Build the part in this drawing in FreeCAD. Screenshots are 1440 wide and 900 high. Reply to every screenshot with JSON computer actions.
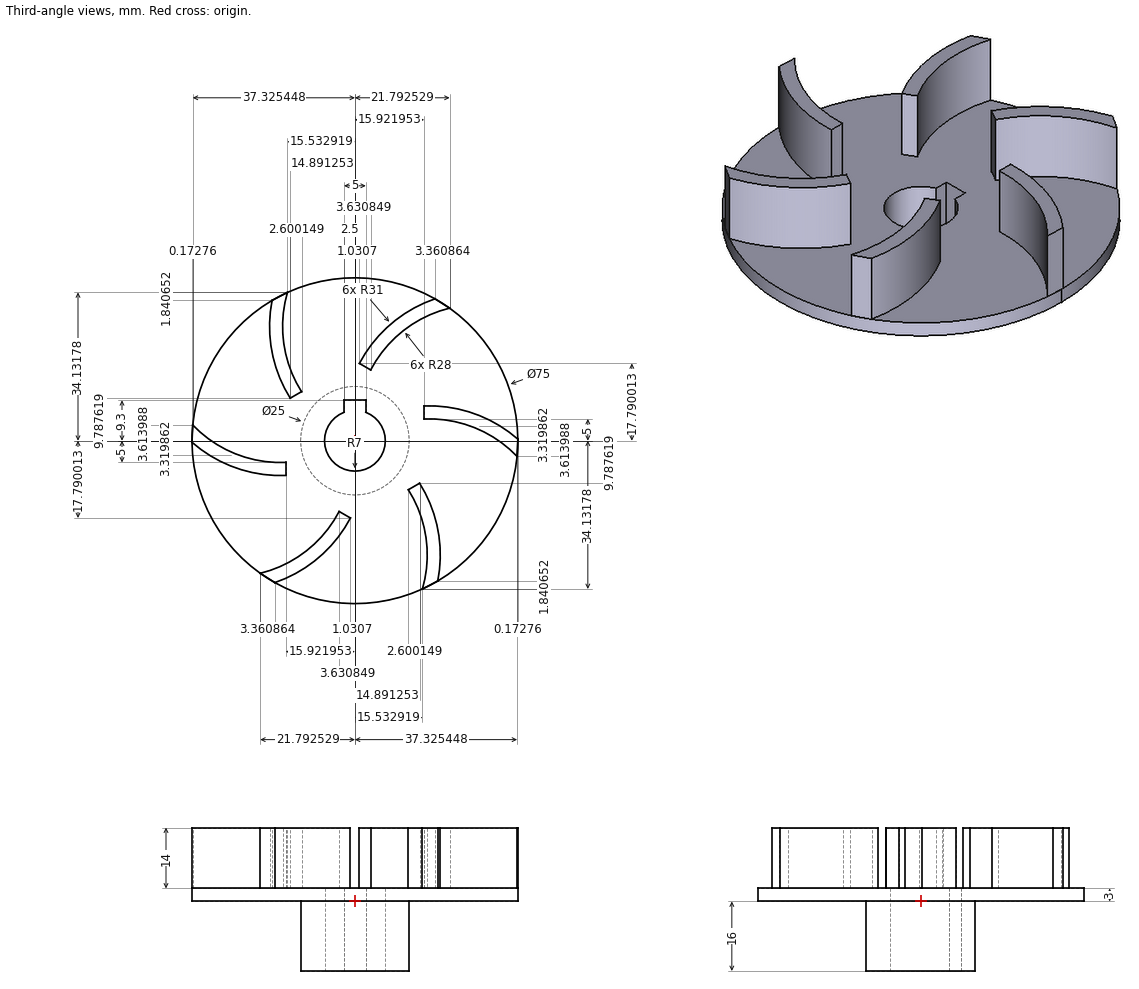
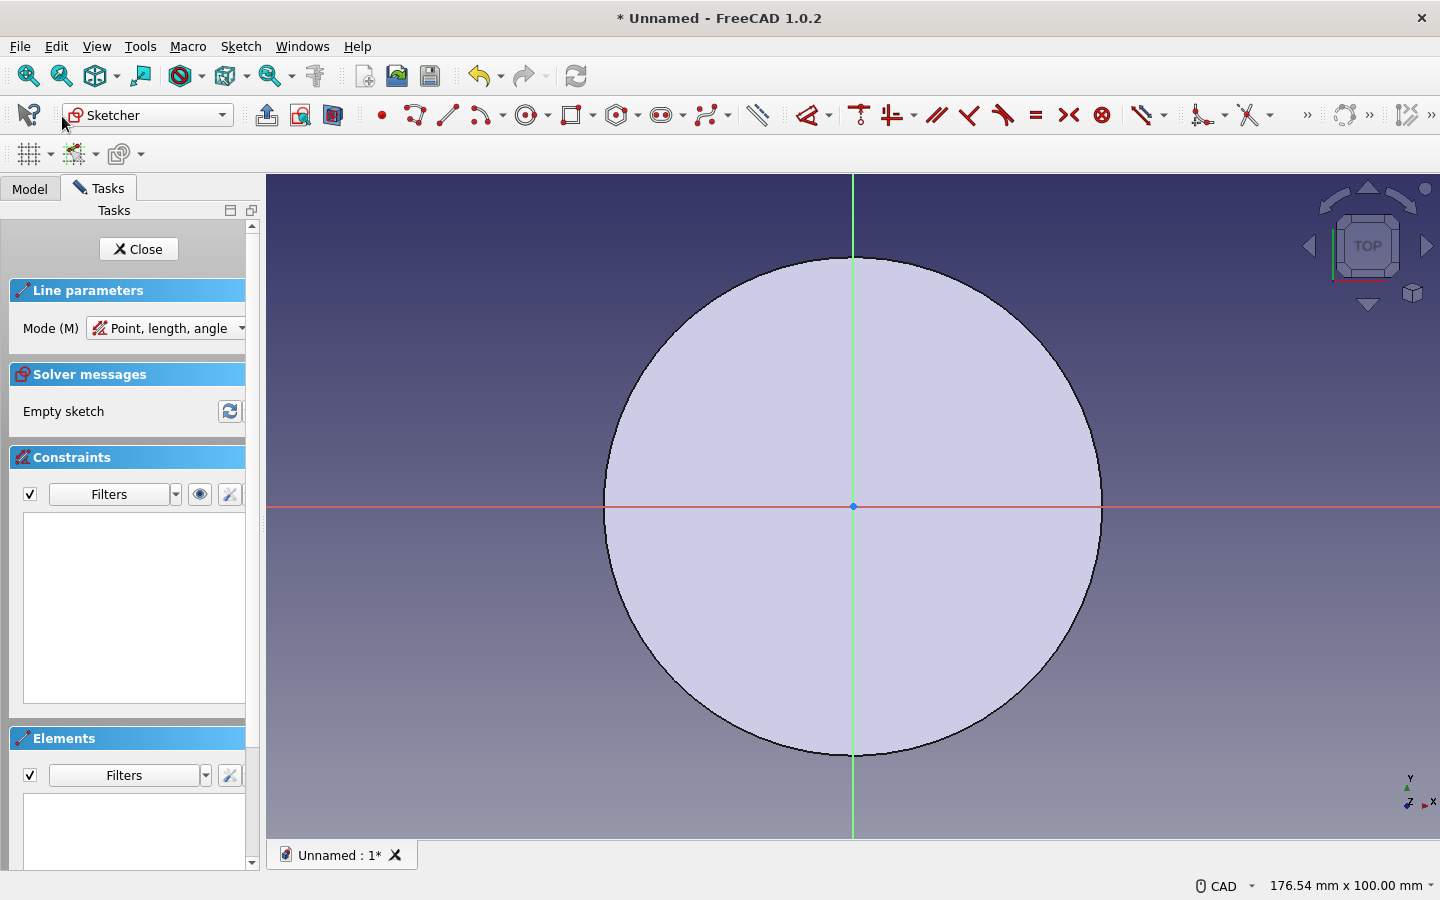
{"action": "left_click", "coordinate": [998, 304]}
{"action": "left_click", "coordinate": [976, 289]}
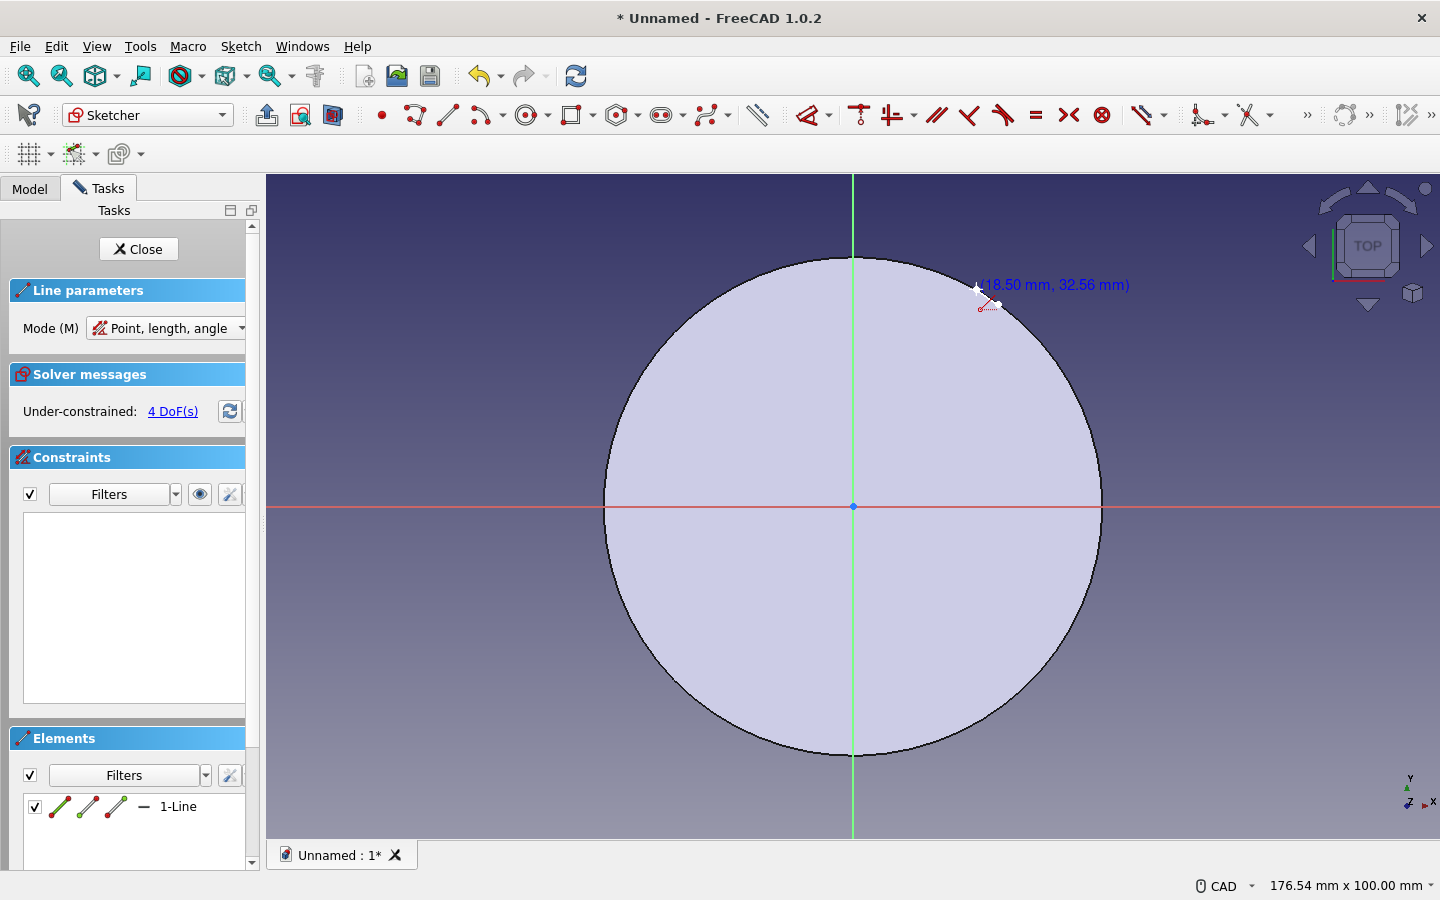
{"action": "scroll", "coordinate": [860, 388], "scroll_direction": "up", "scroll_amount": 5}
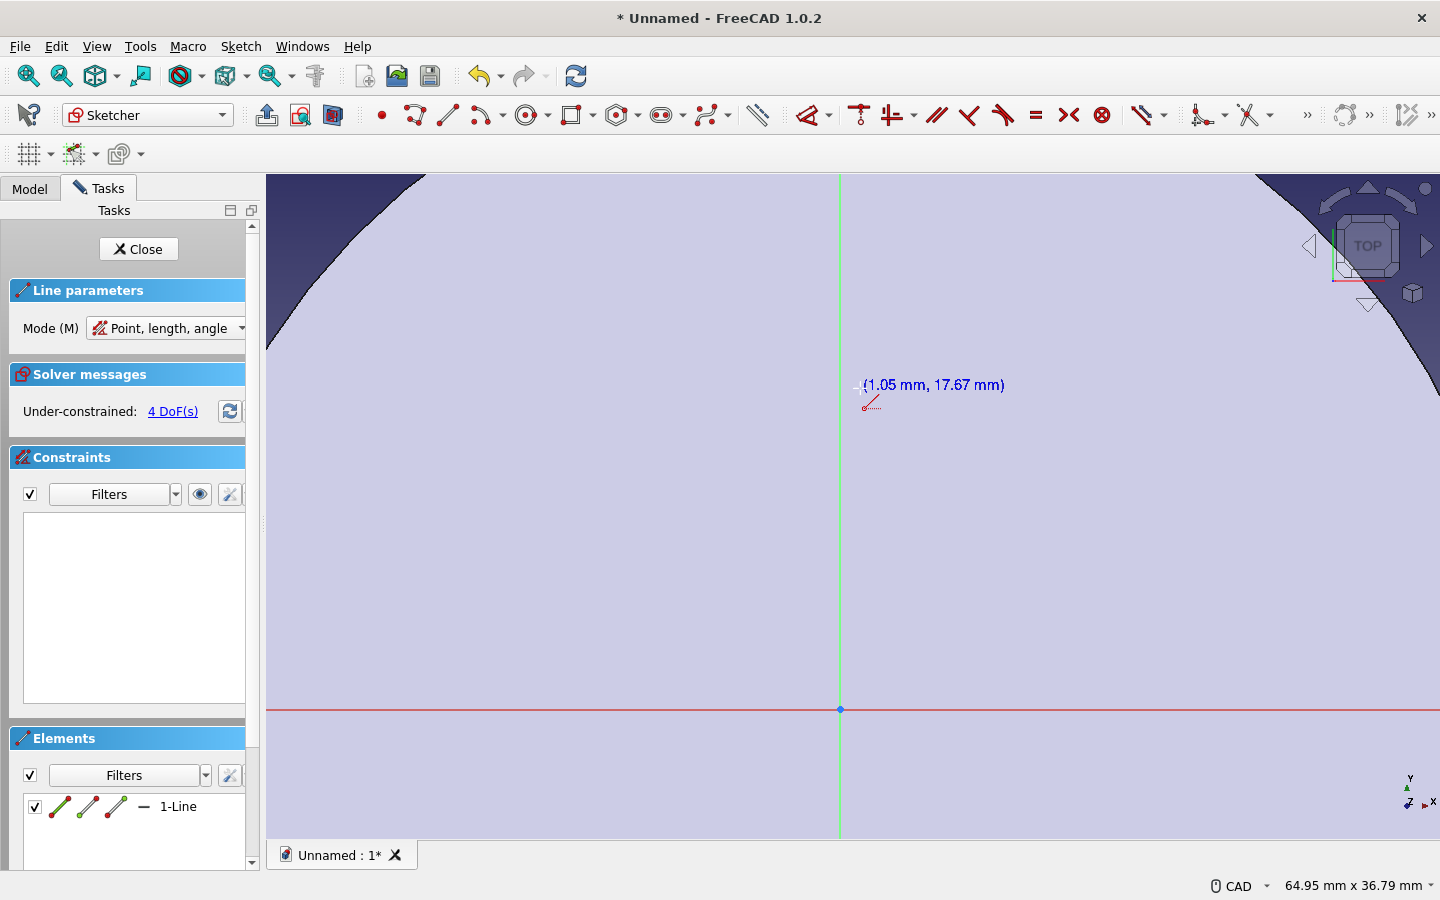
{"action": "left_click", "coordinate": [859, 388]}
{"action": "left_click", "coordinate": [906, 415]}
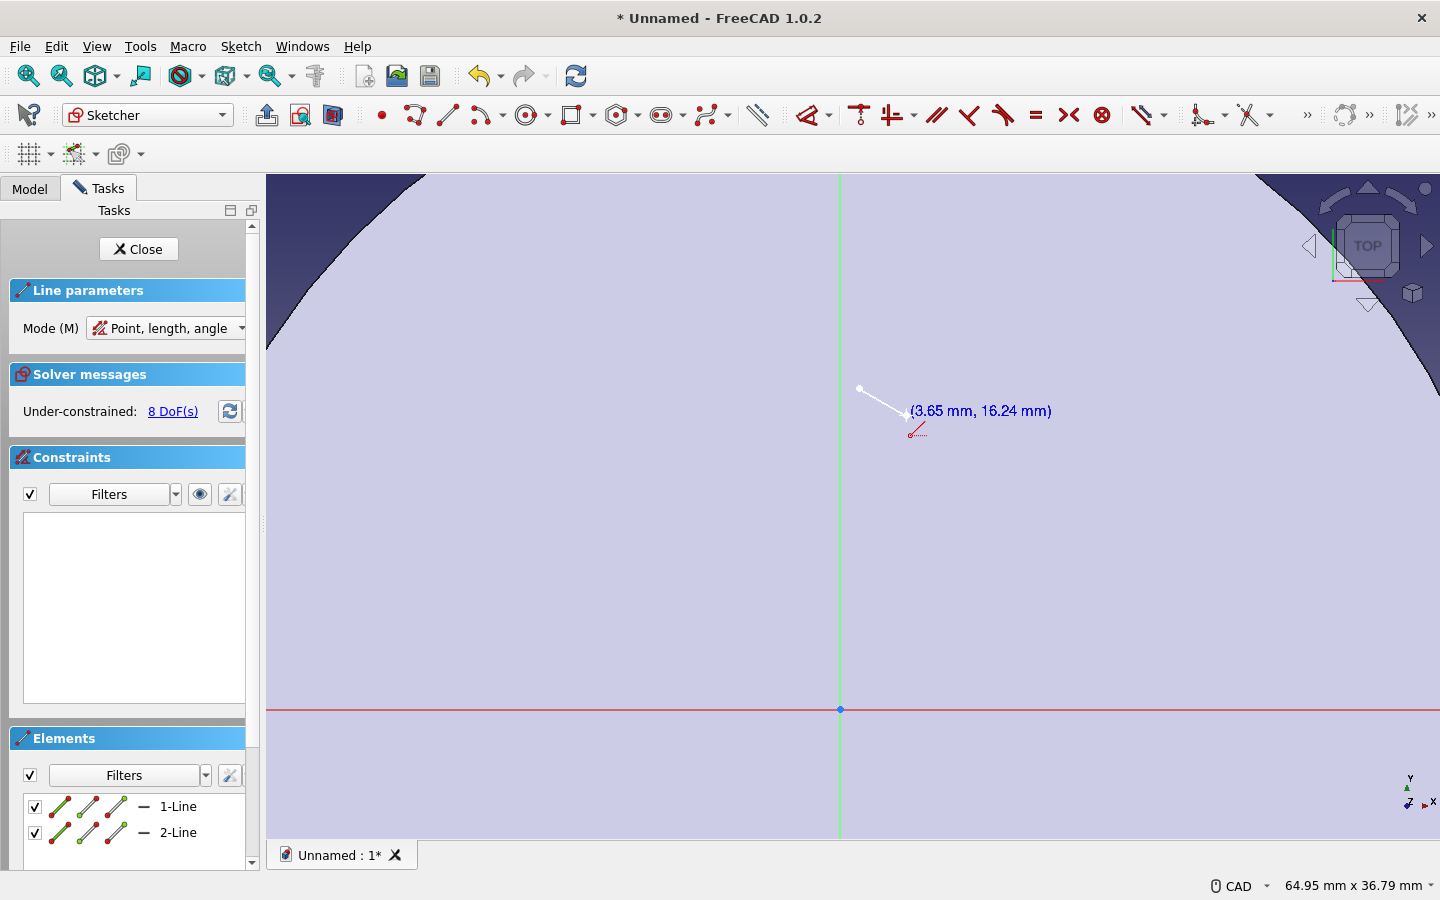
{"action": "key", "text": "g 3 a"}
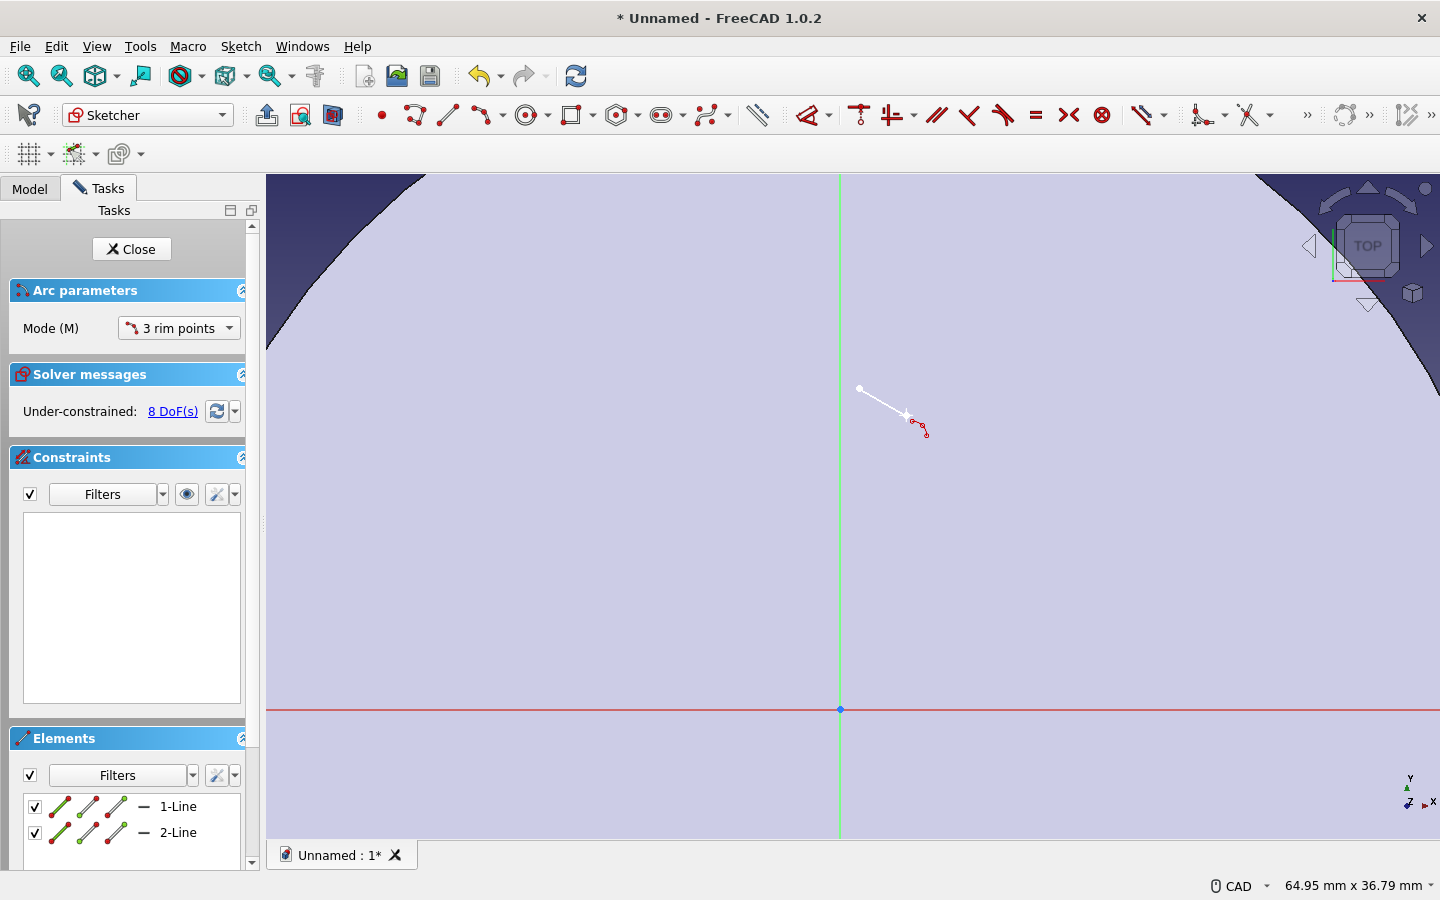
{"action": "scroll", "coordinate": [752, 388], "scroll_direction": "down", "scroll_amount": 5}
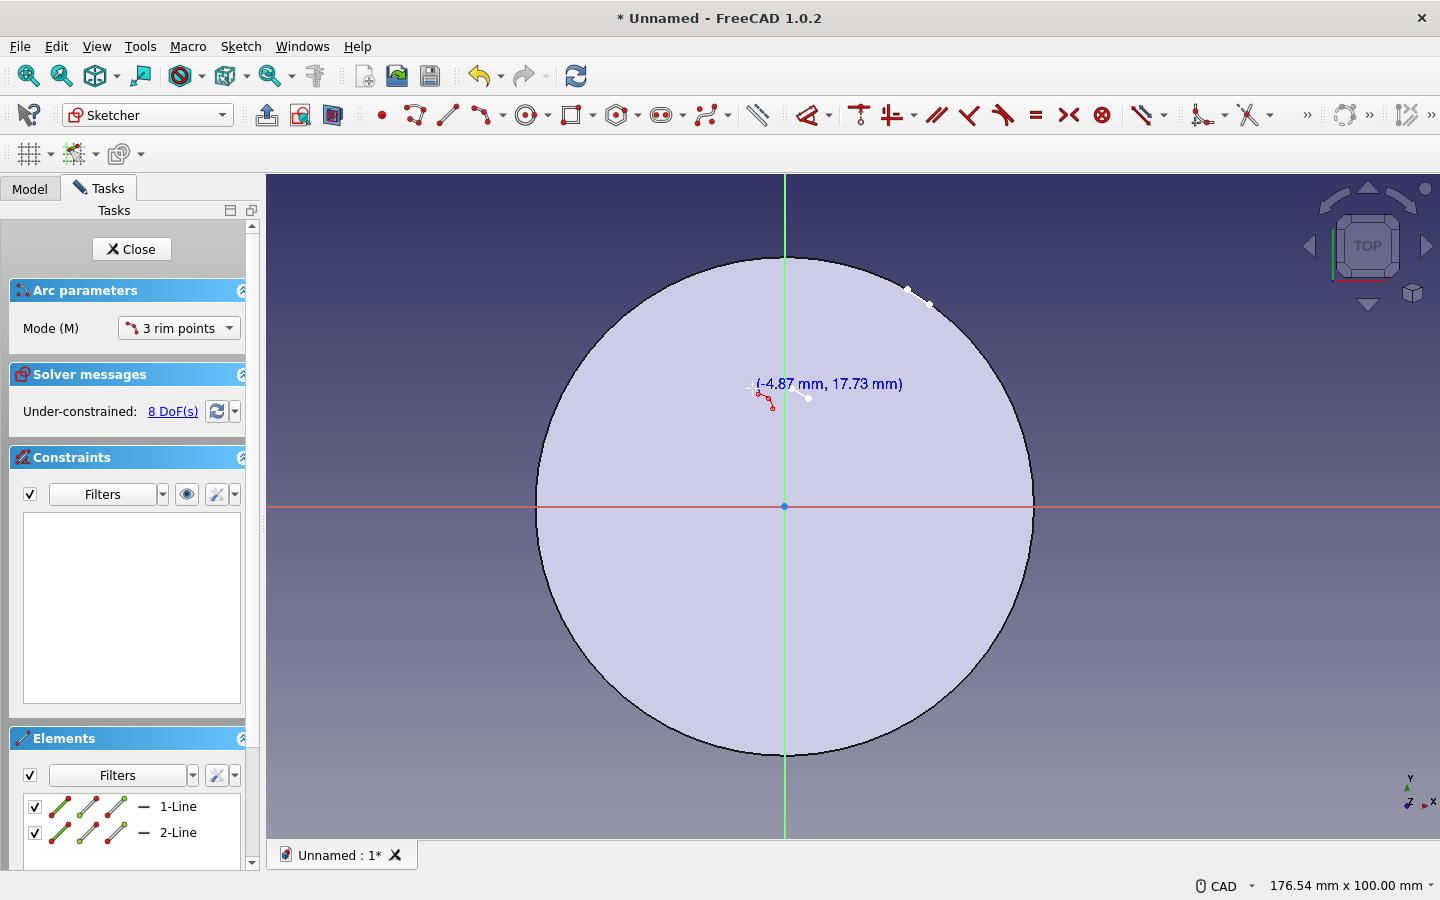
{"action": "left_click", "coordinate": [908, 290]}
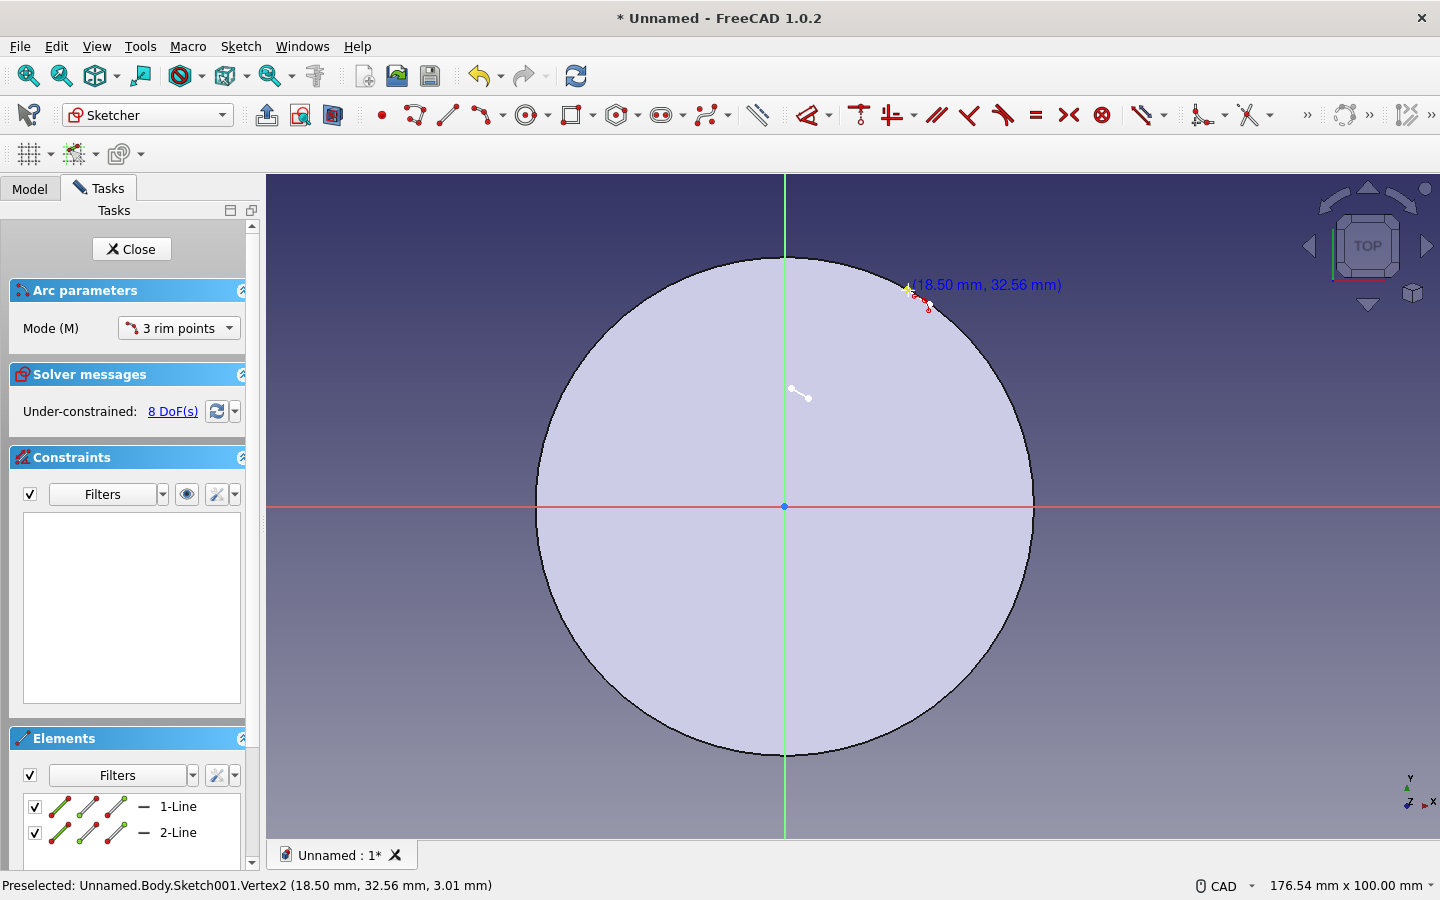
{"action": "scroll", "coordinate": [792, 388], "scroll_direction": "up", "scroll_amount": 5}